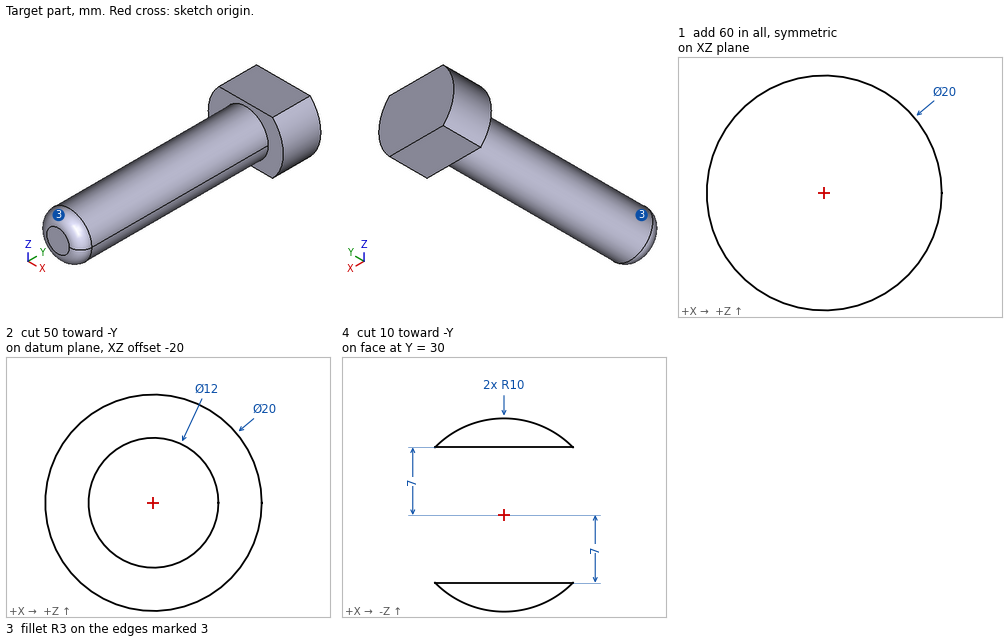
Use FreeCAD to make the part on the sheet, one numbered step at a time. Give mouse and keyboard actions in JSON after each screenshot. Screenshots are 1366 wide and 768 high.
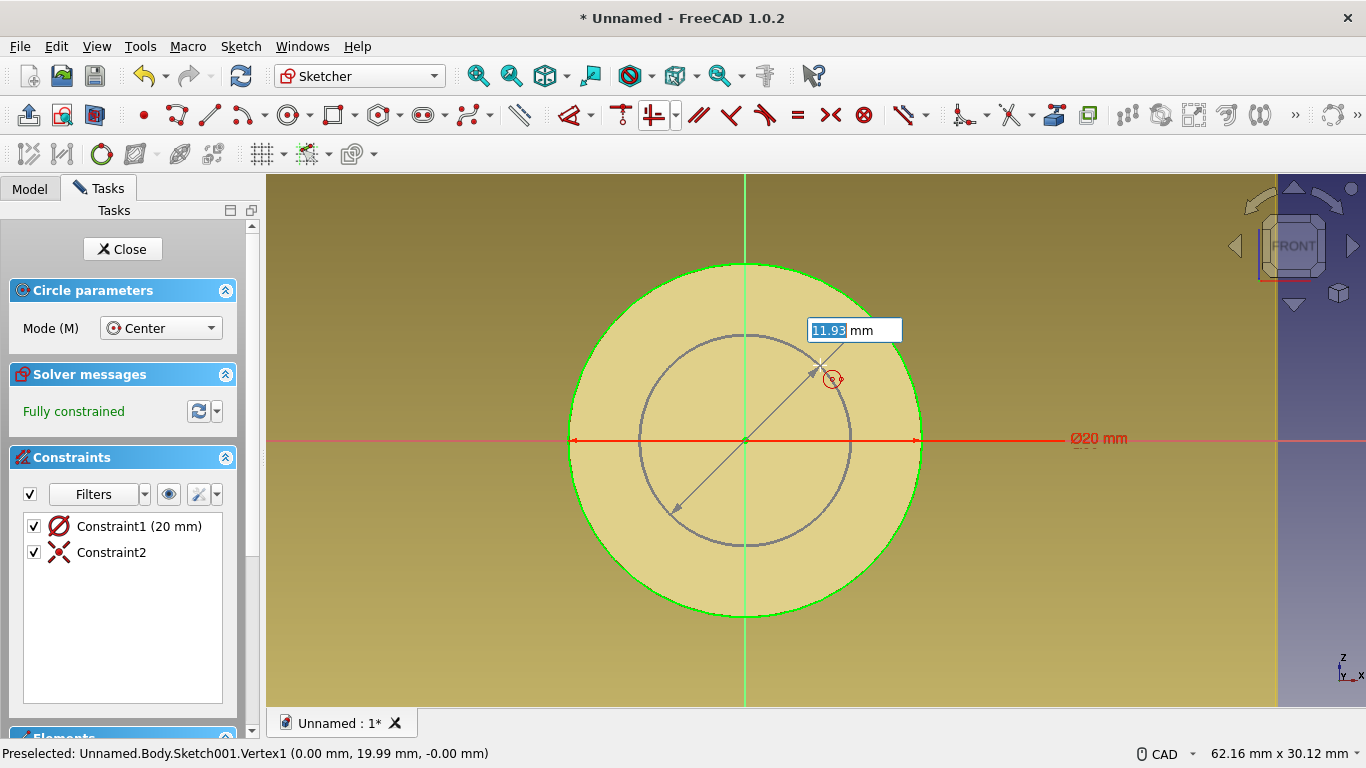
{"action": "type", "text": "12"}
{"action": "key", "text": "Return"}
{"action": "key", "text": "Escape"}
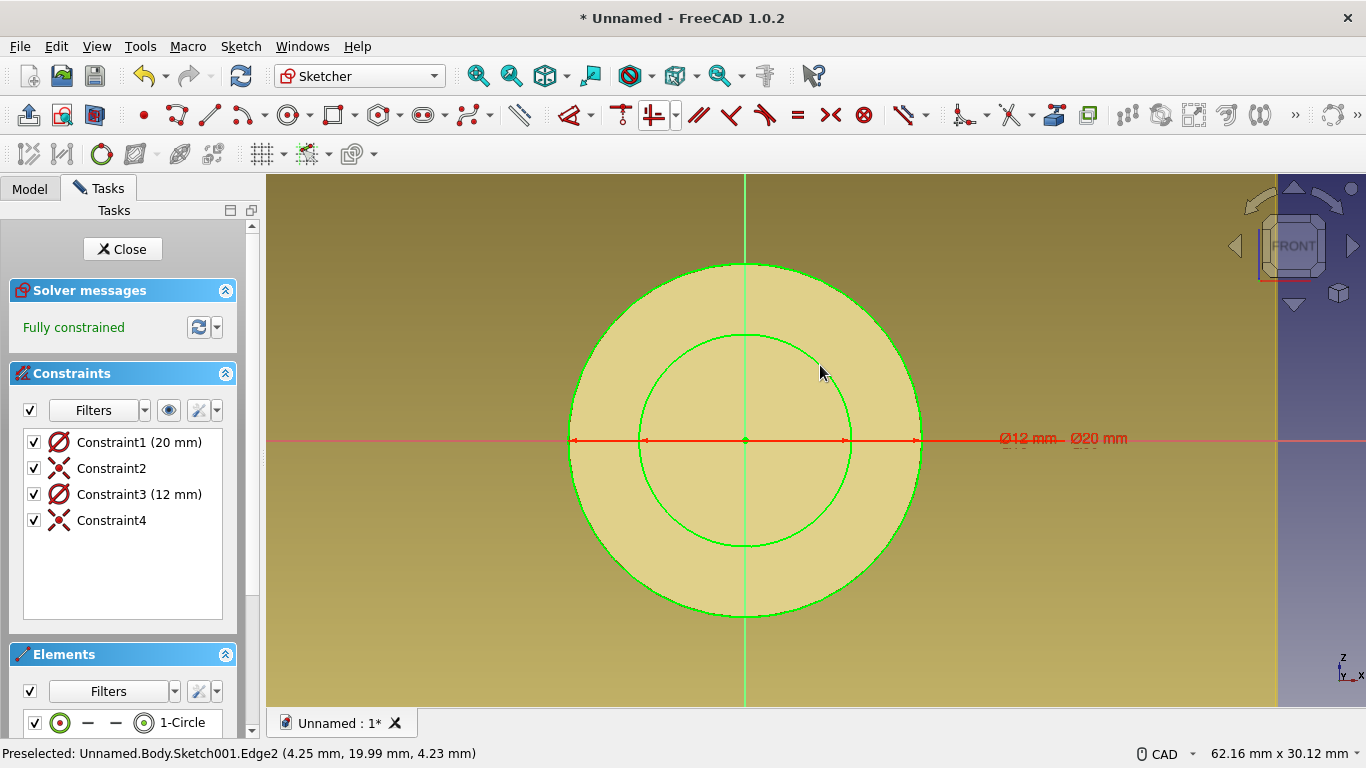
{"action": "left_click", "coordinate": [123, 249]}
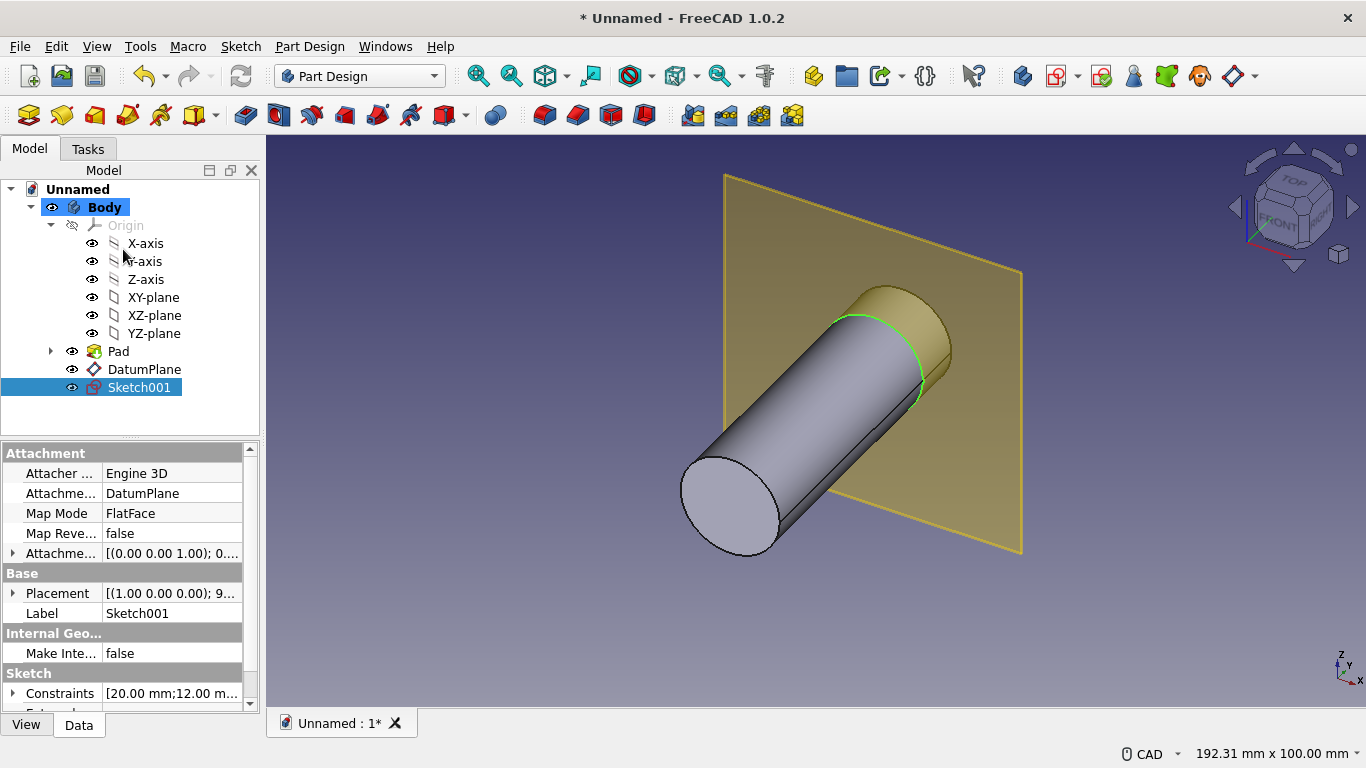
{"action": "left_click", "coordinate": [246, 116]}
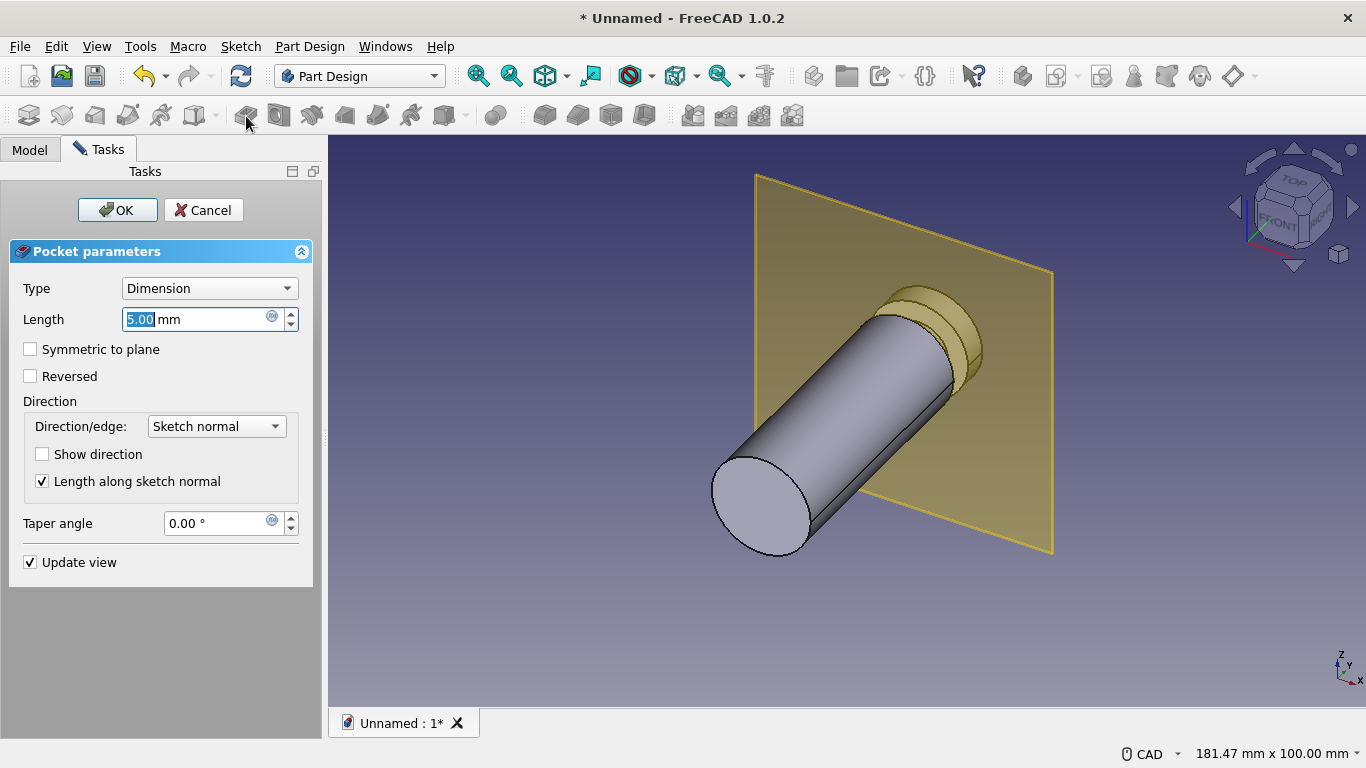
{"action": "type", "text": "50"}
{"action": "key", "text": "Tab"}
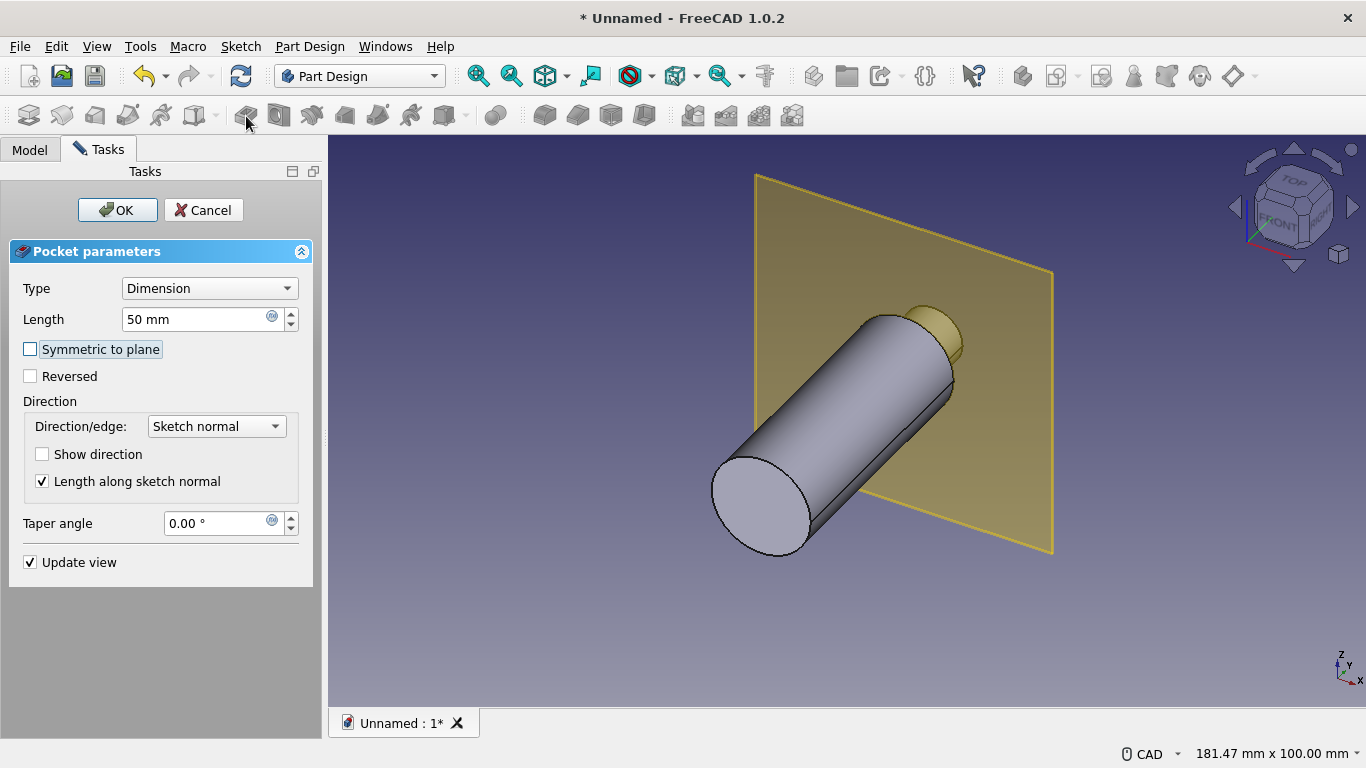
{"action": "left_click", "coordinate": [31, 376]}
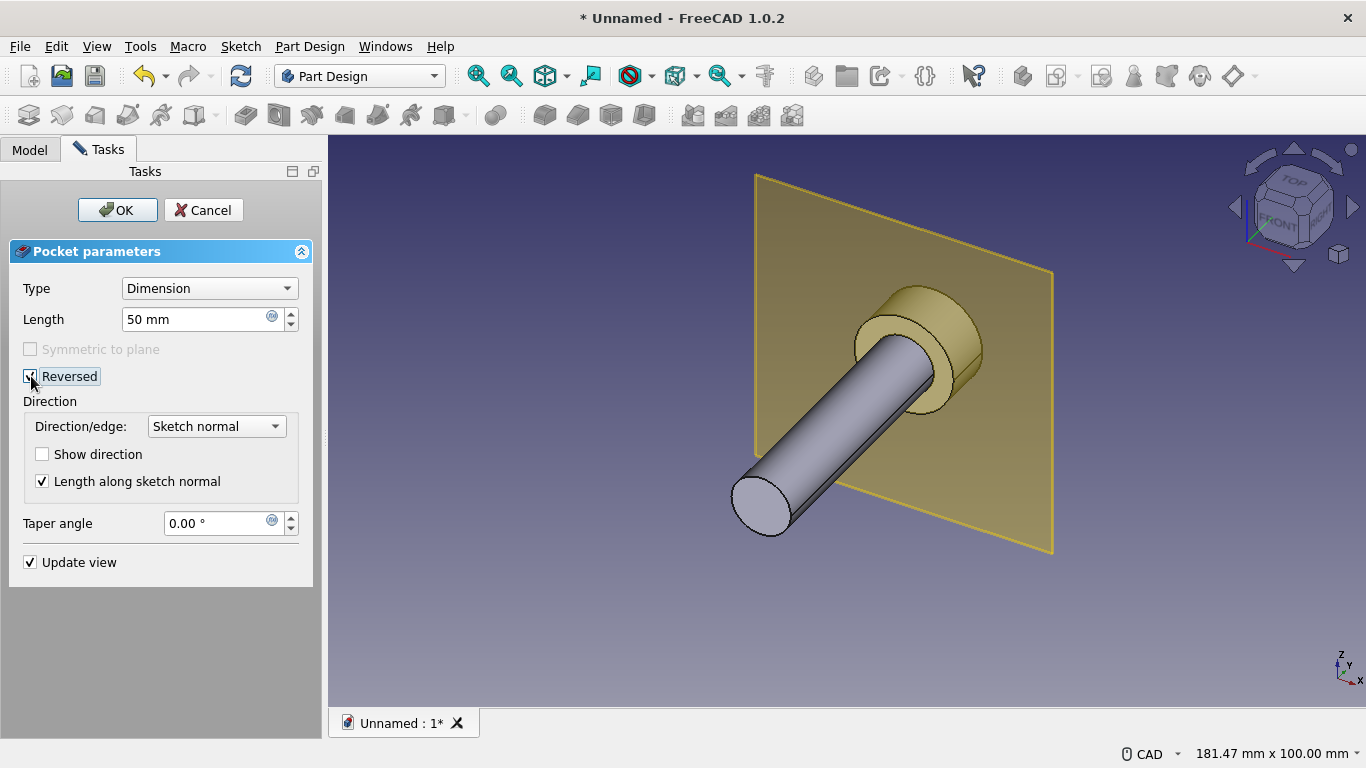
{"action": "left_click", "coordinate": [118, 210]}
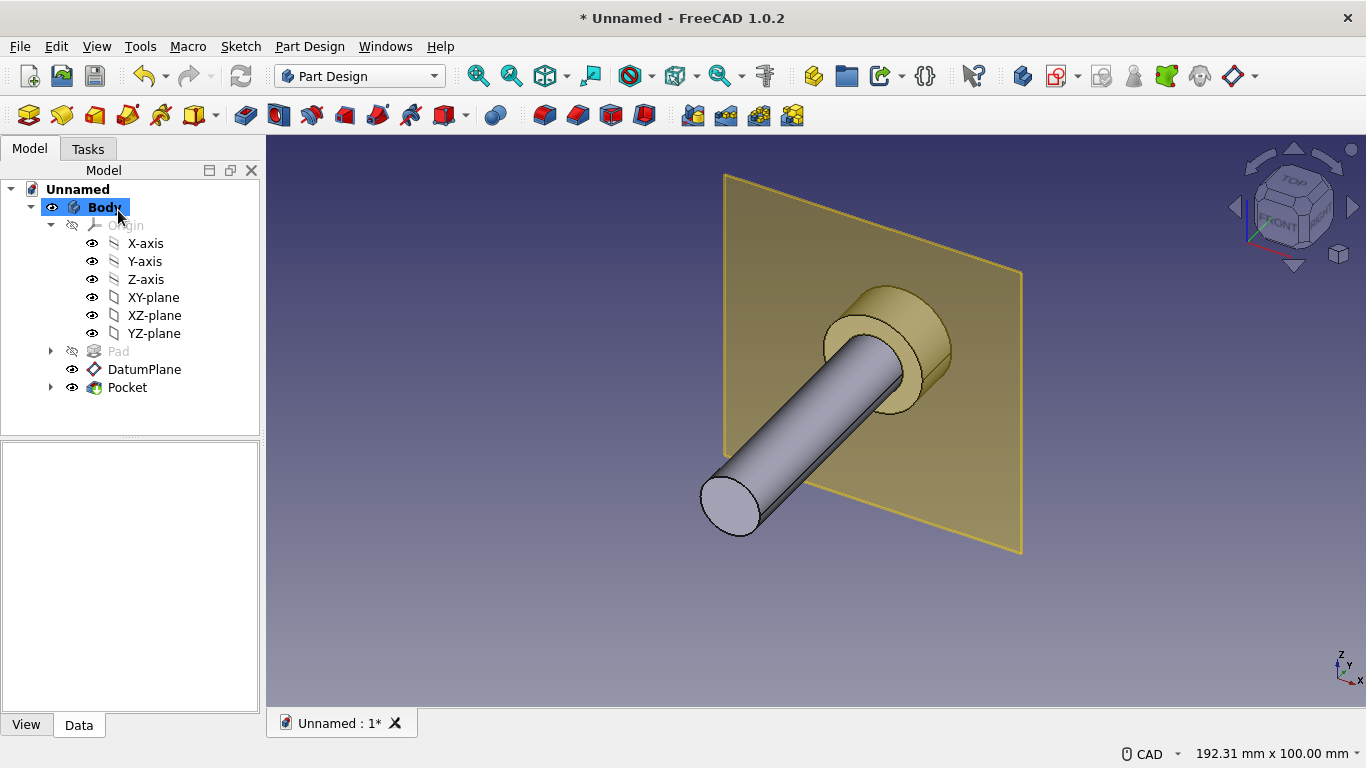
{"action": "left_click", "coordinate": [117, 369]}
{"action": "key", "text": "space"}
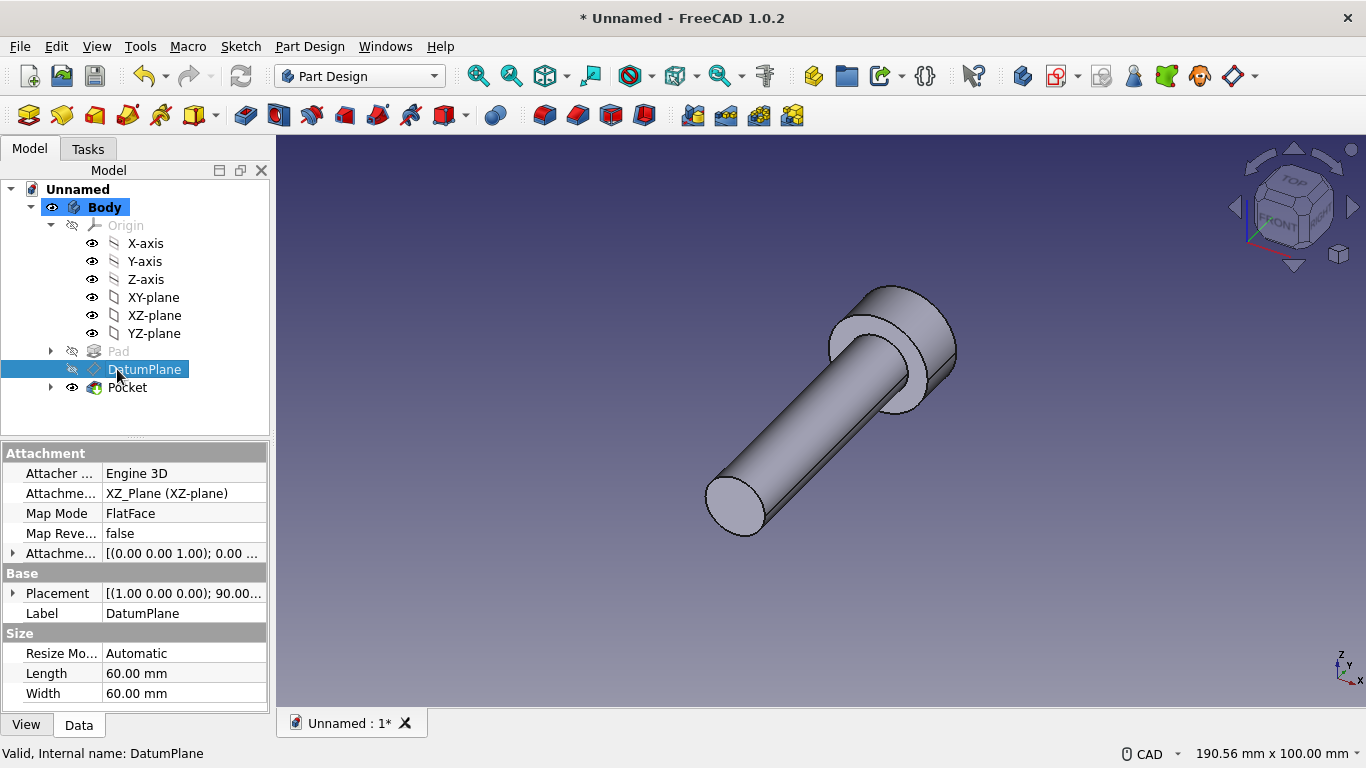
{"action": "left_click", "coordinate": [711, 481]}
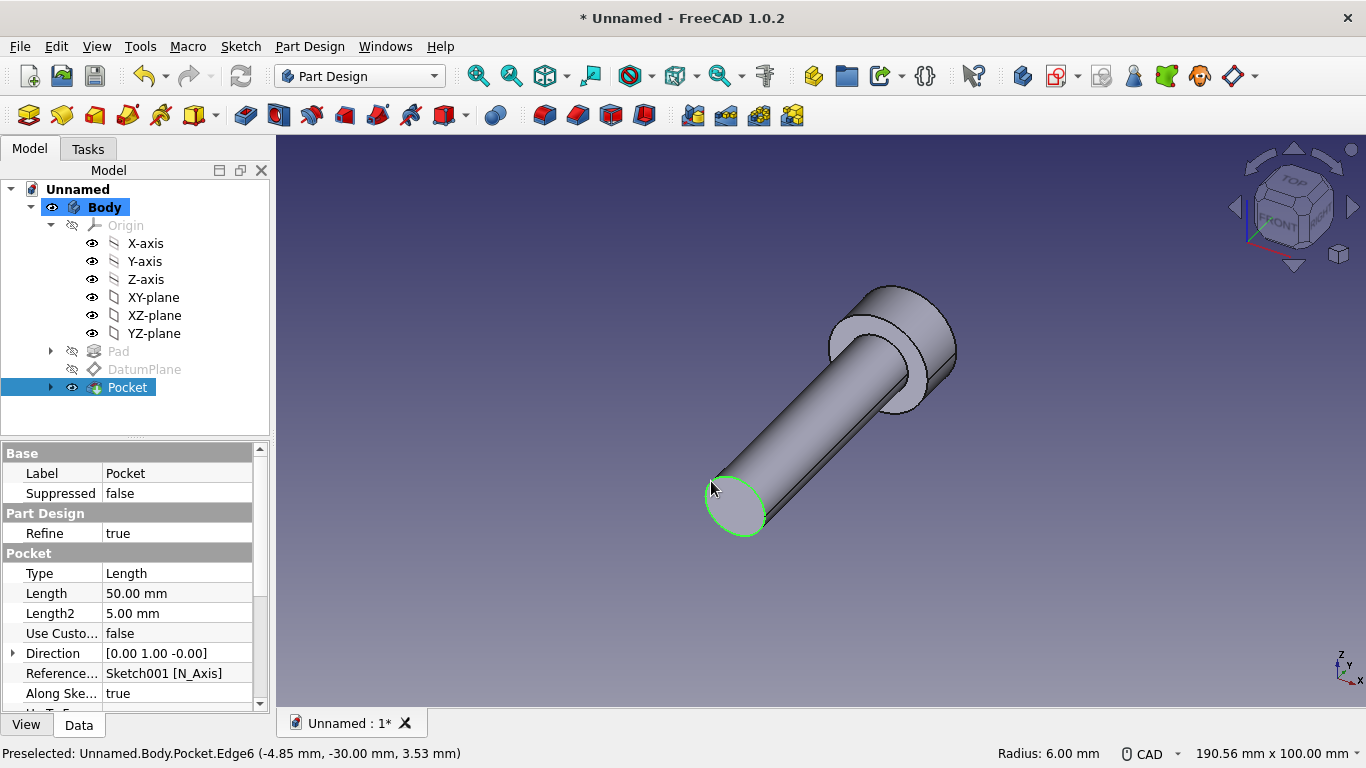
{"action": "left_click", "coordinate": [545, 116]}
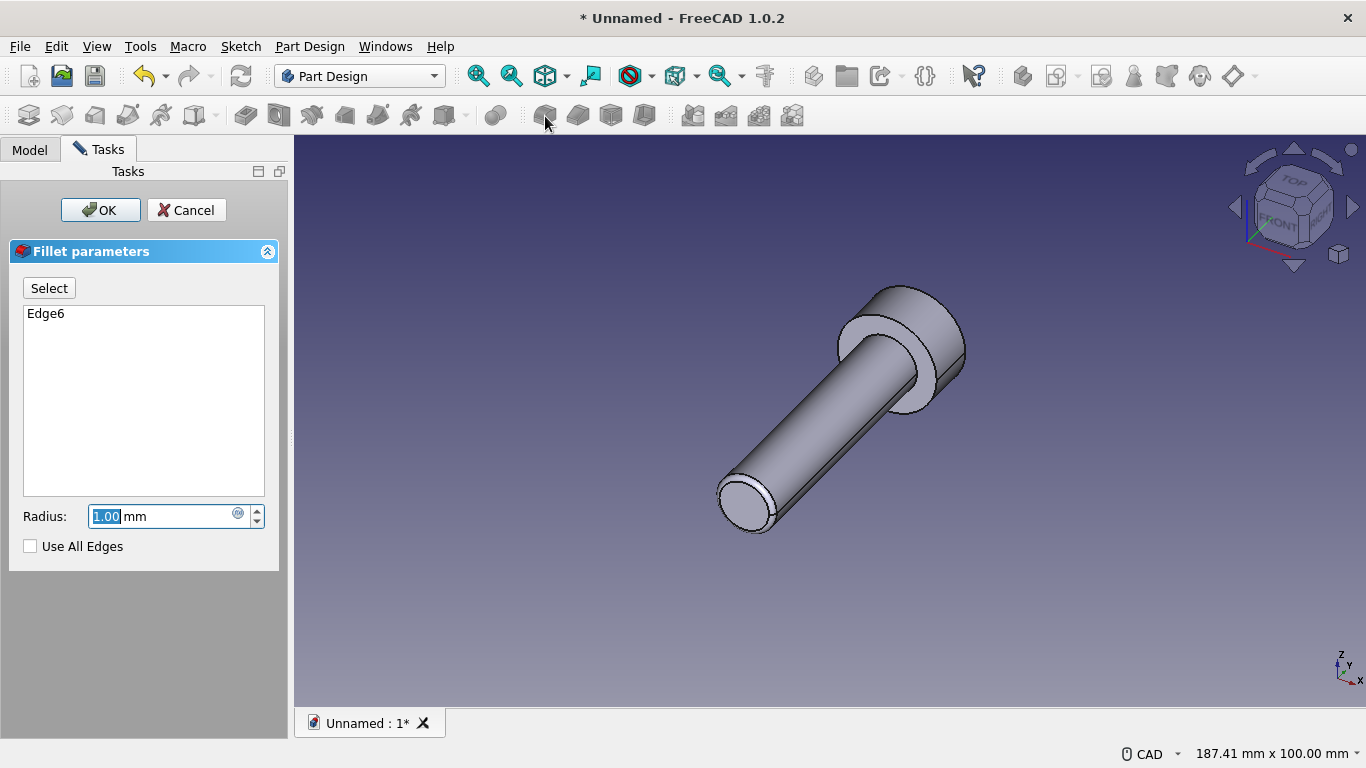
{"action": "type", "text": "3"}
{"action": "key", "text": "Tab"}